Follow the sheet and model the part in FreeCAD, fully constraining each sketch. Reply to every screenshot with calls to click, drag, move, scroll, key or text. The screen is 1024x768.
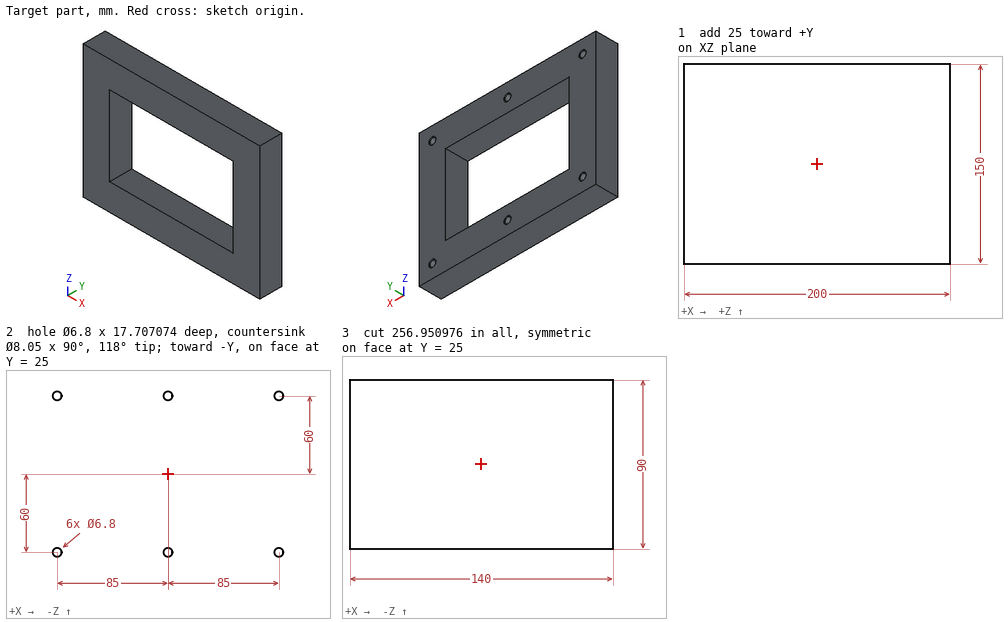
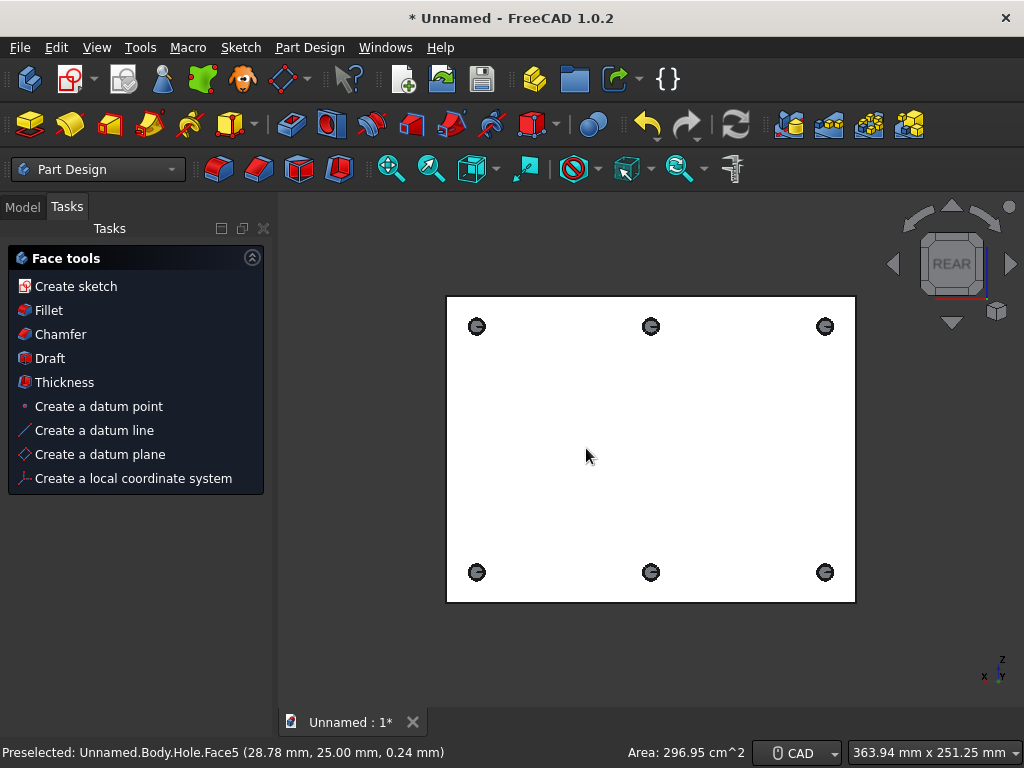
click(70, 80)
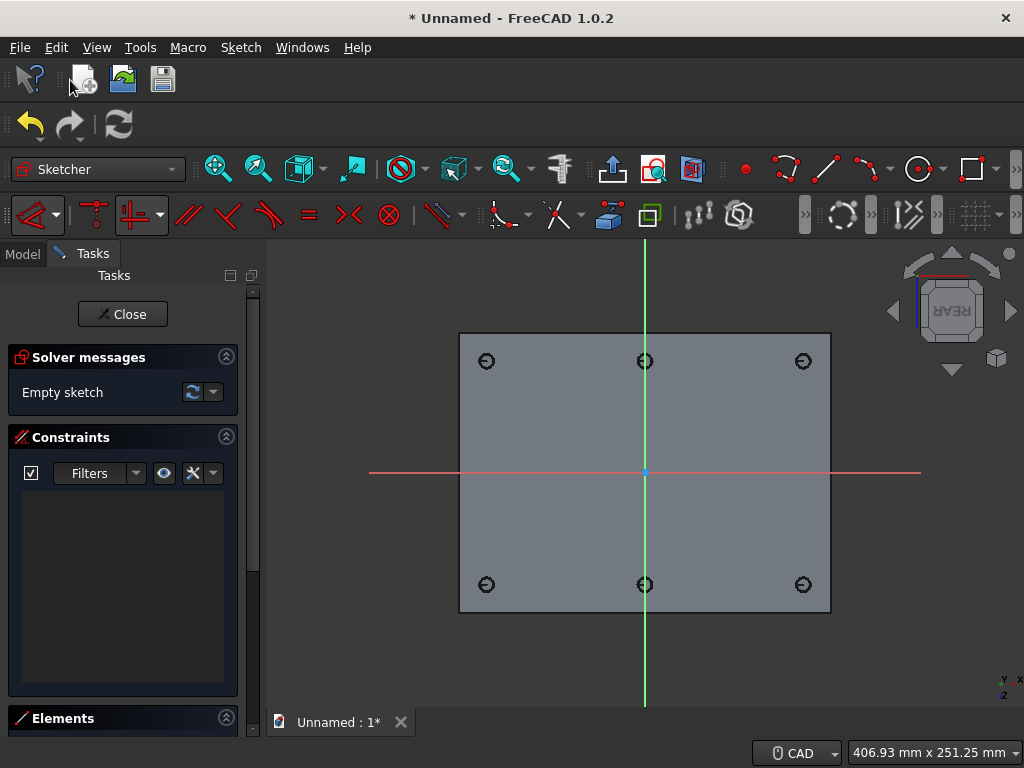
scroll(784, 473, up, 2)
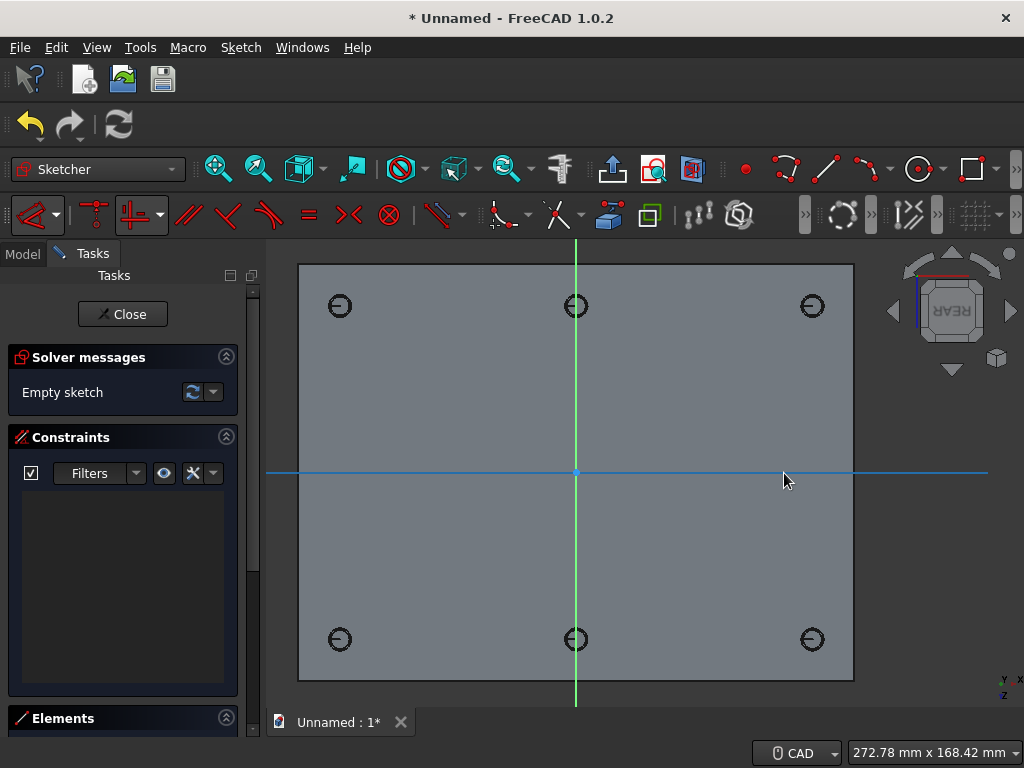
key(g)
key(v)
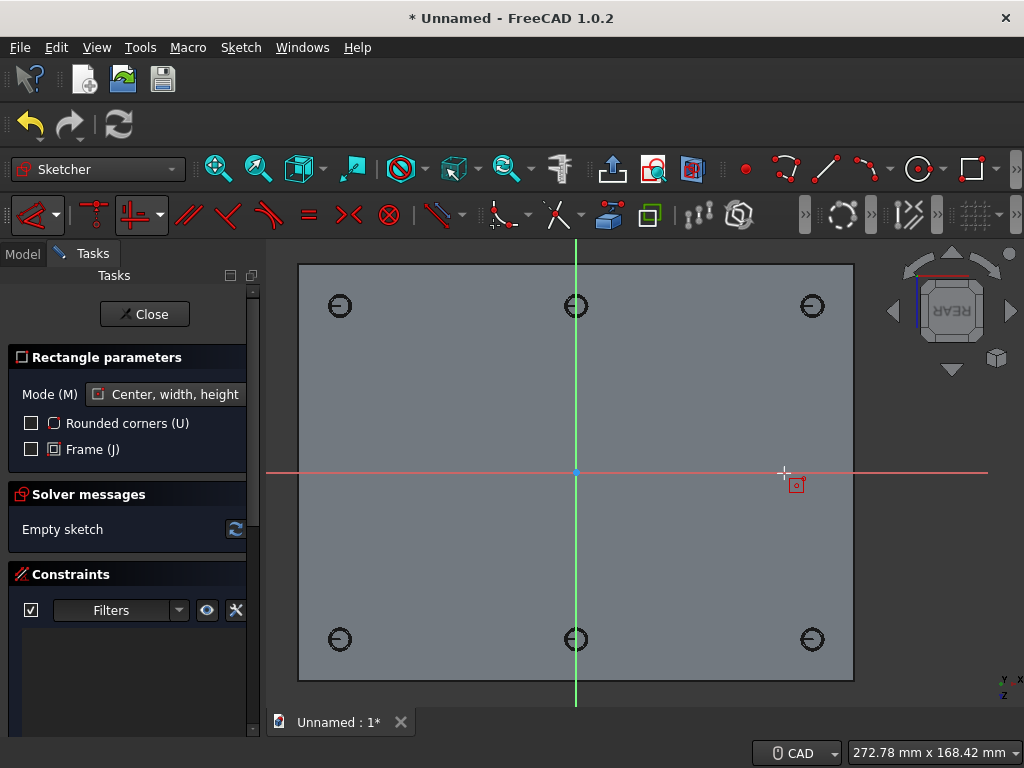
click(576, 473)
click(771, 348)
key(Escape)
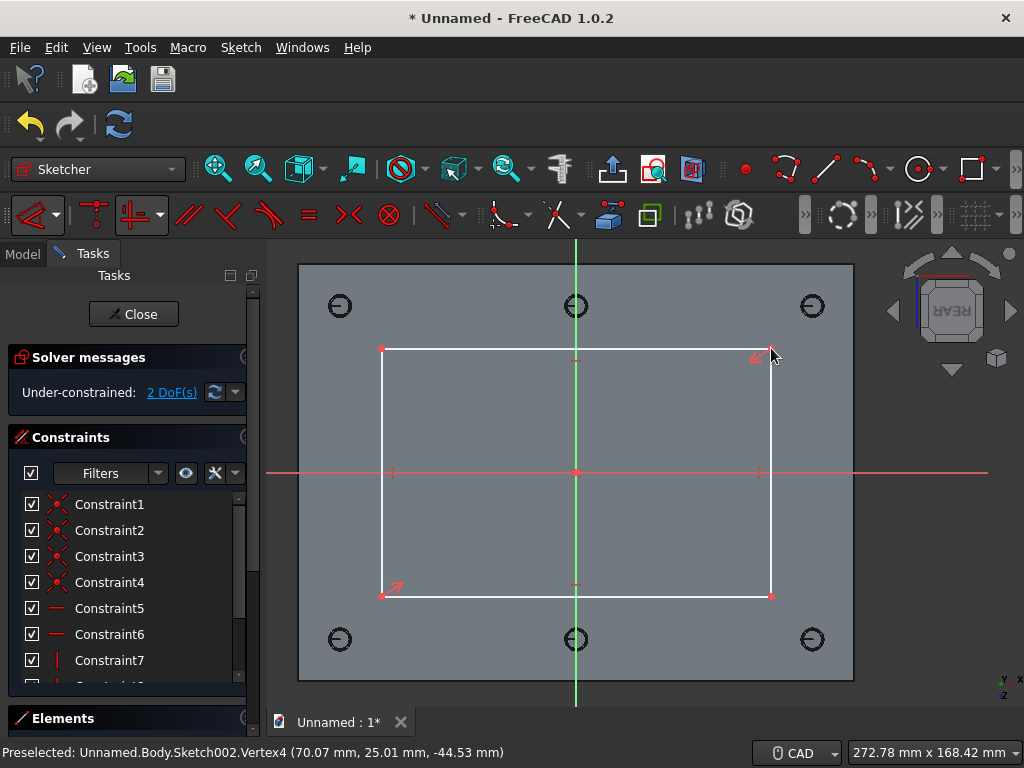
click(771, 522)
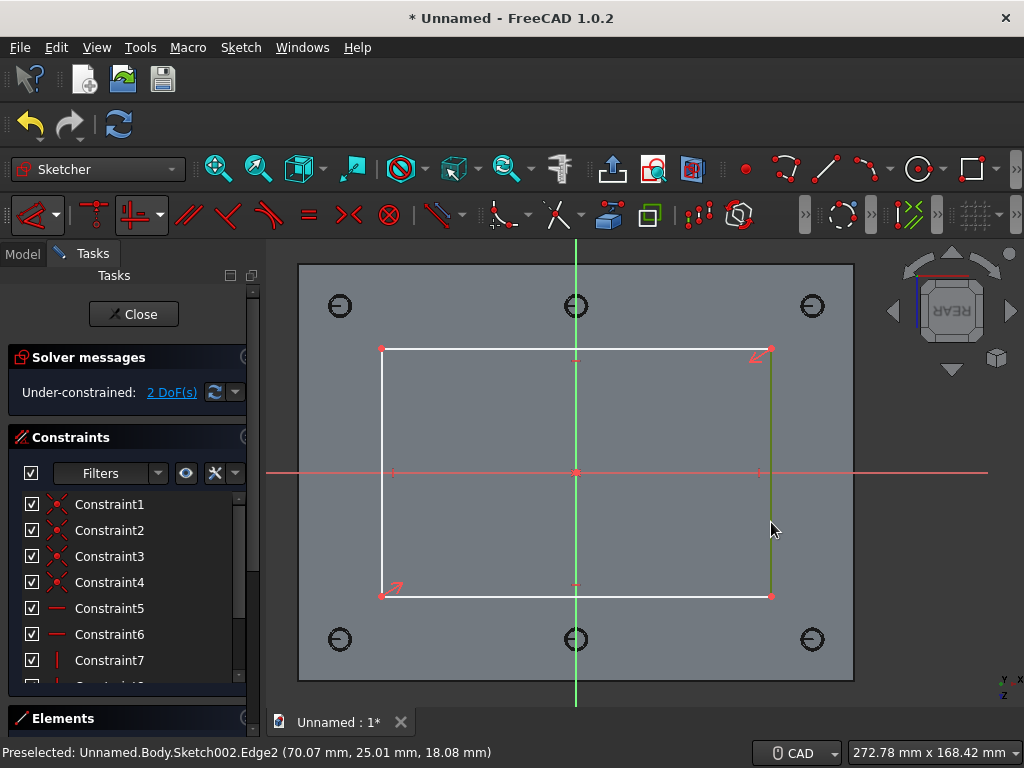
key(i)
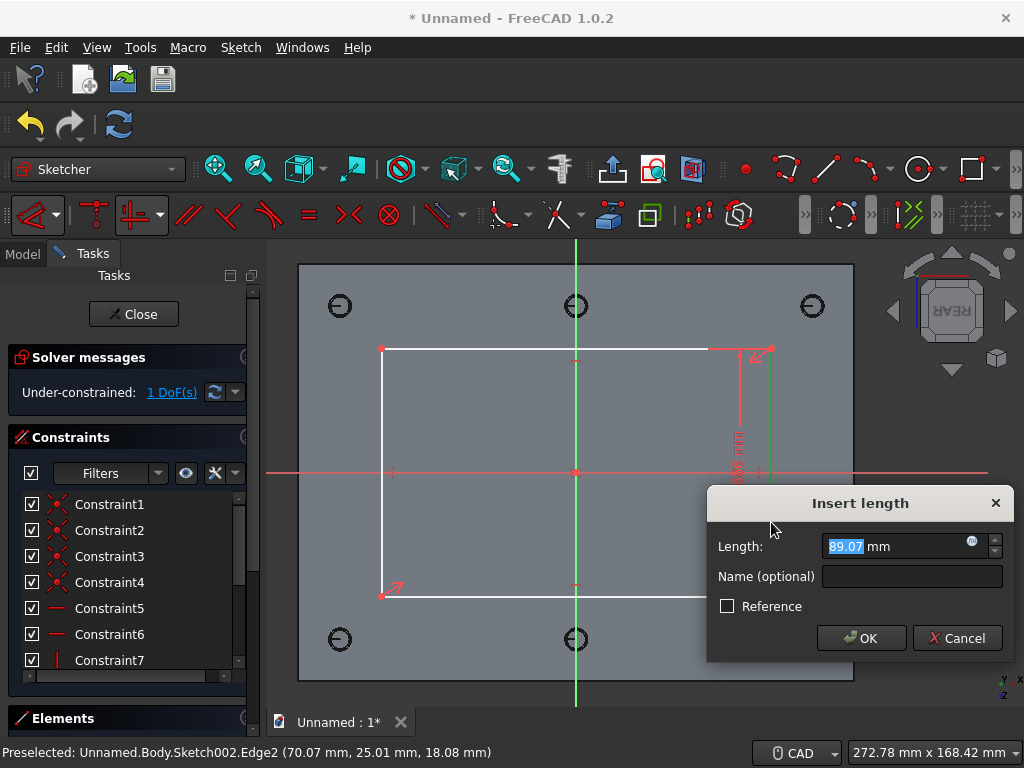
text(90)
key(Return)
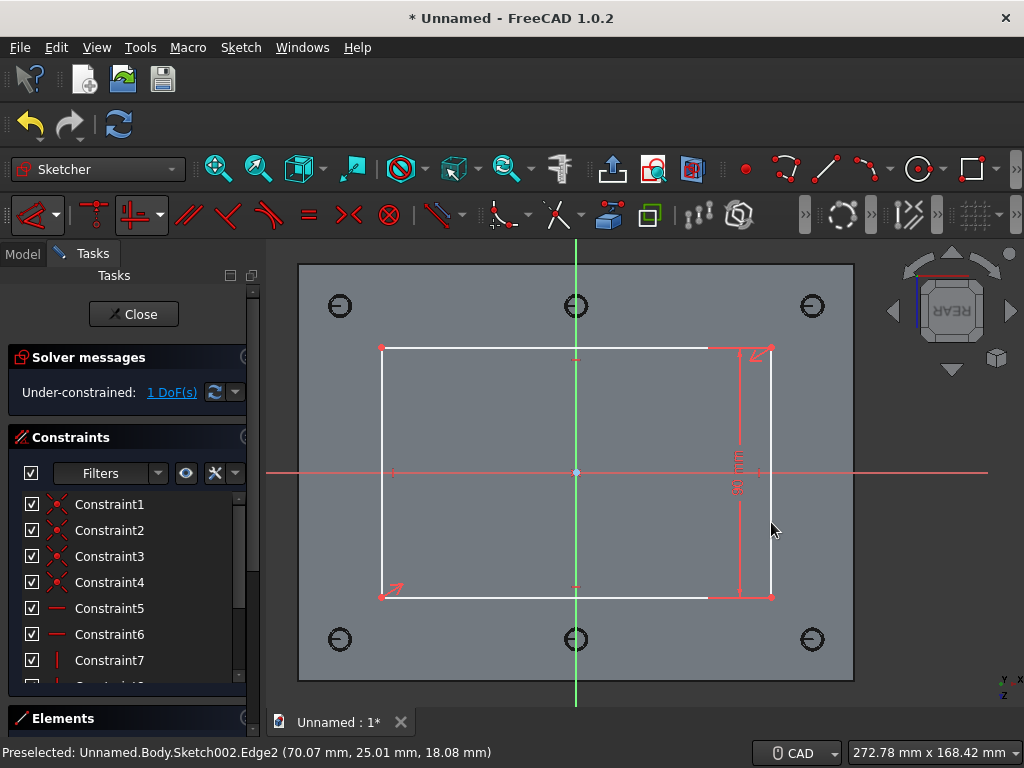
click(498, 598)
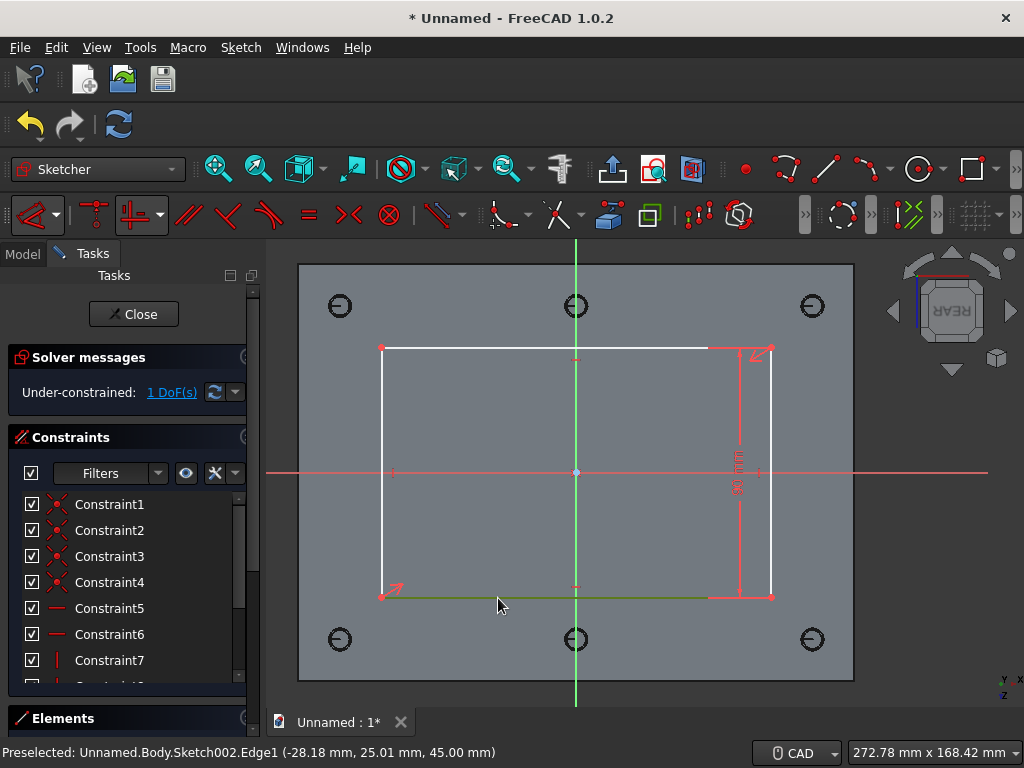
click(58, 216)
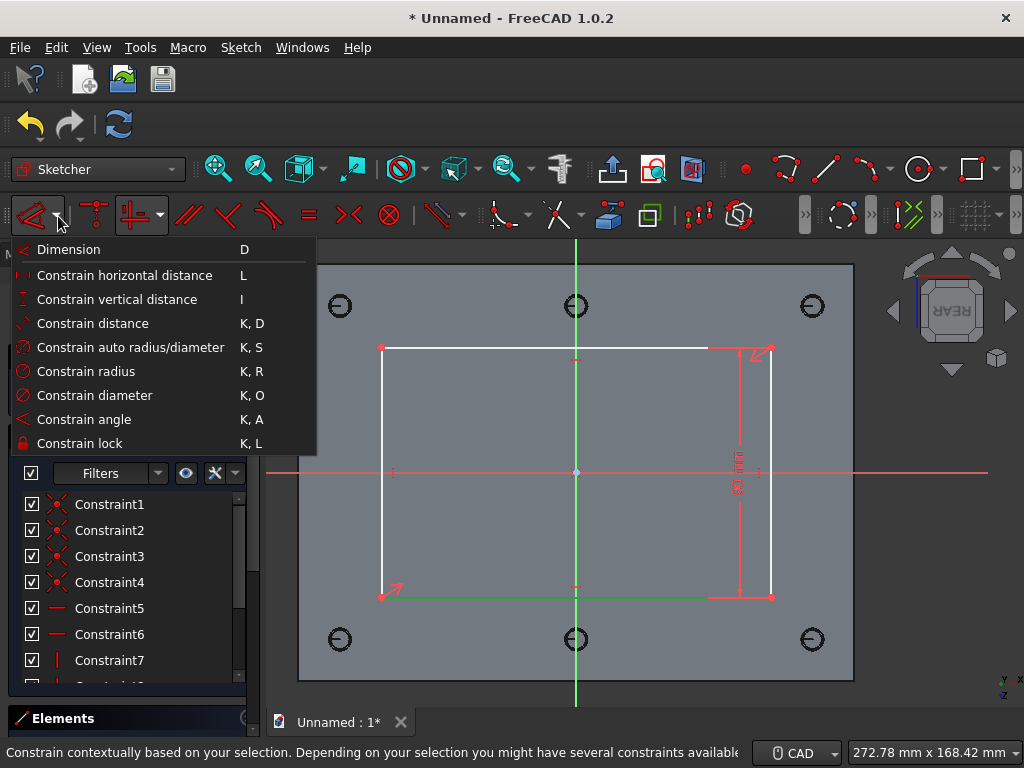
click(164, 275)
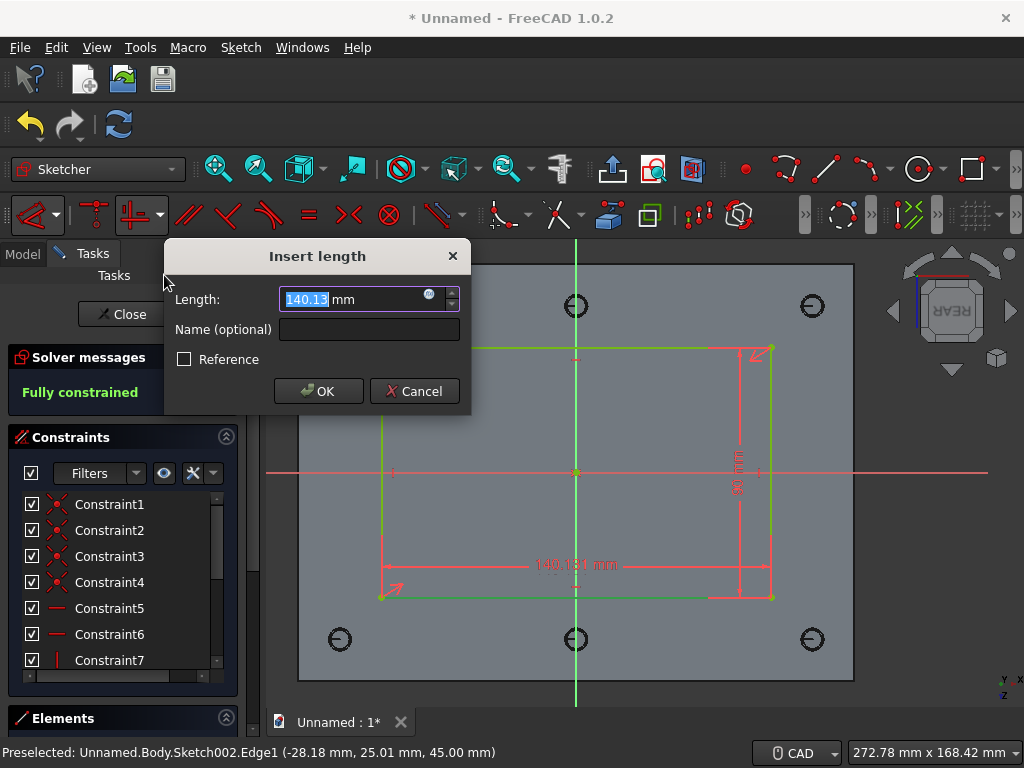
text(140)
key(Return)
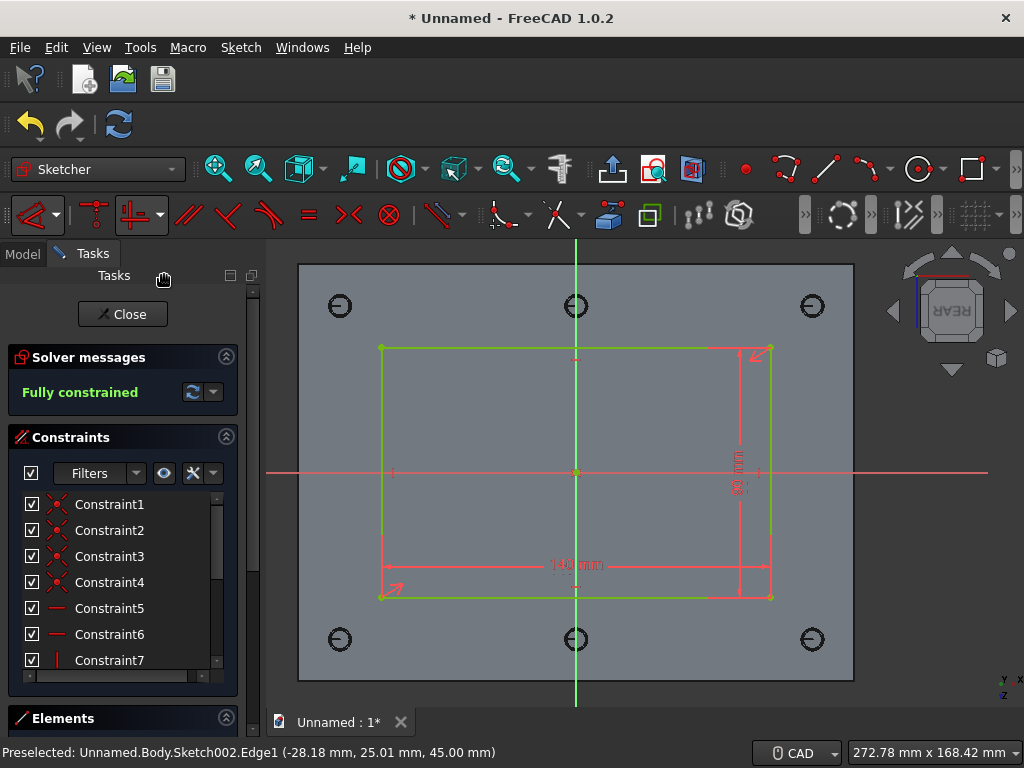
click(123, 314)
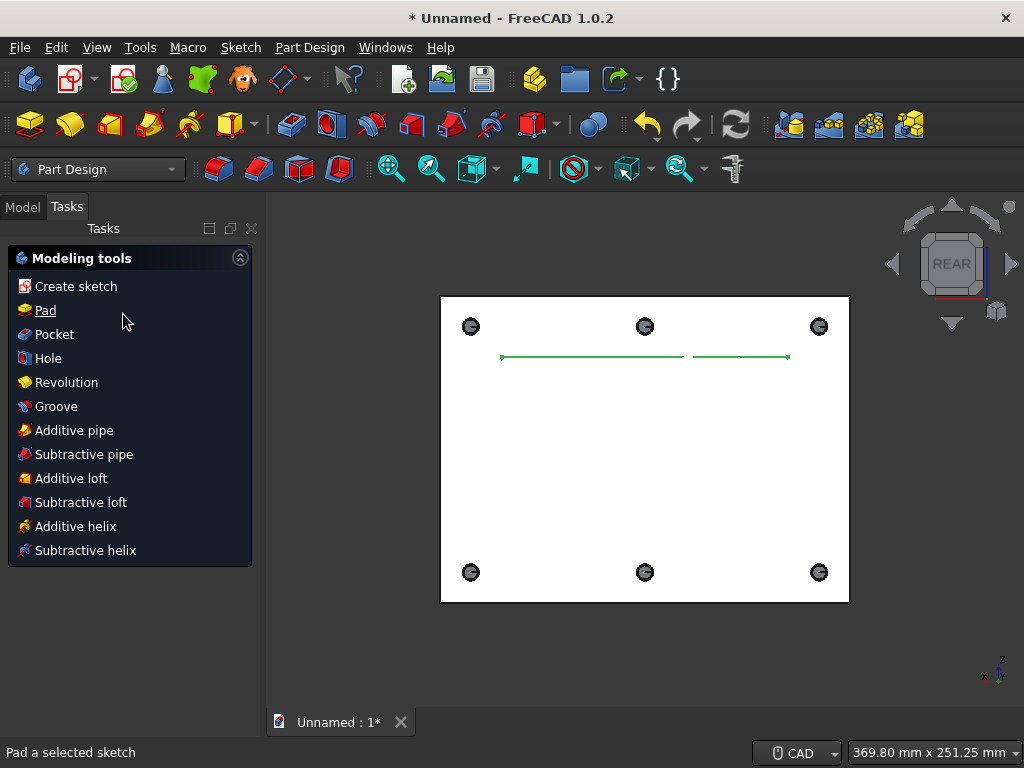
click(292, 124)